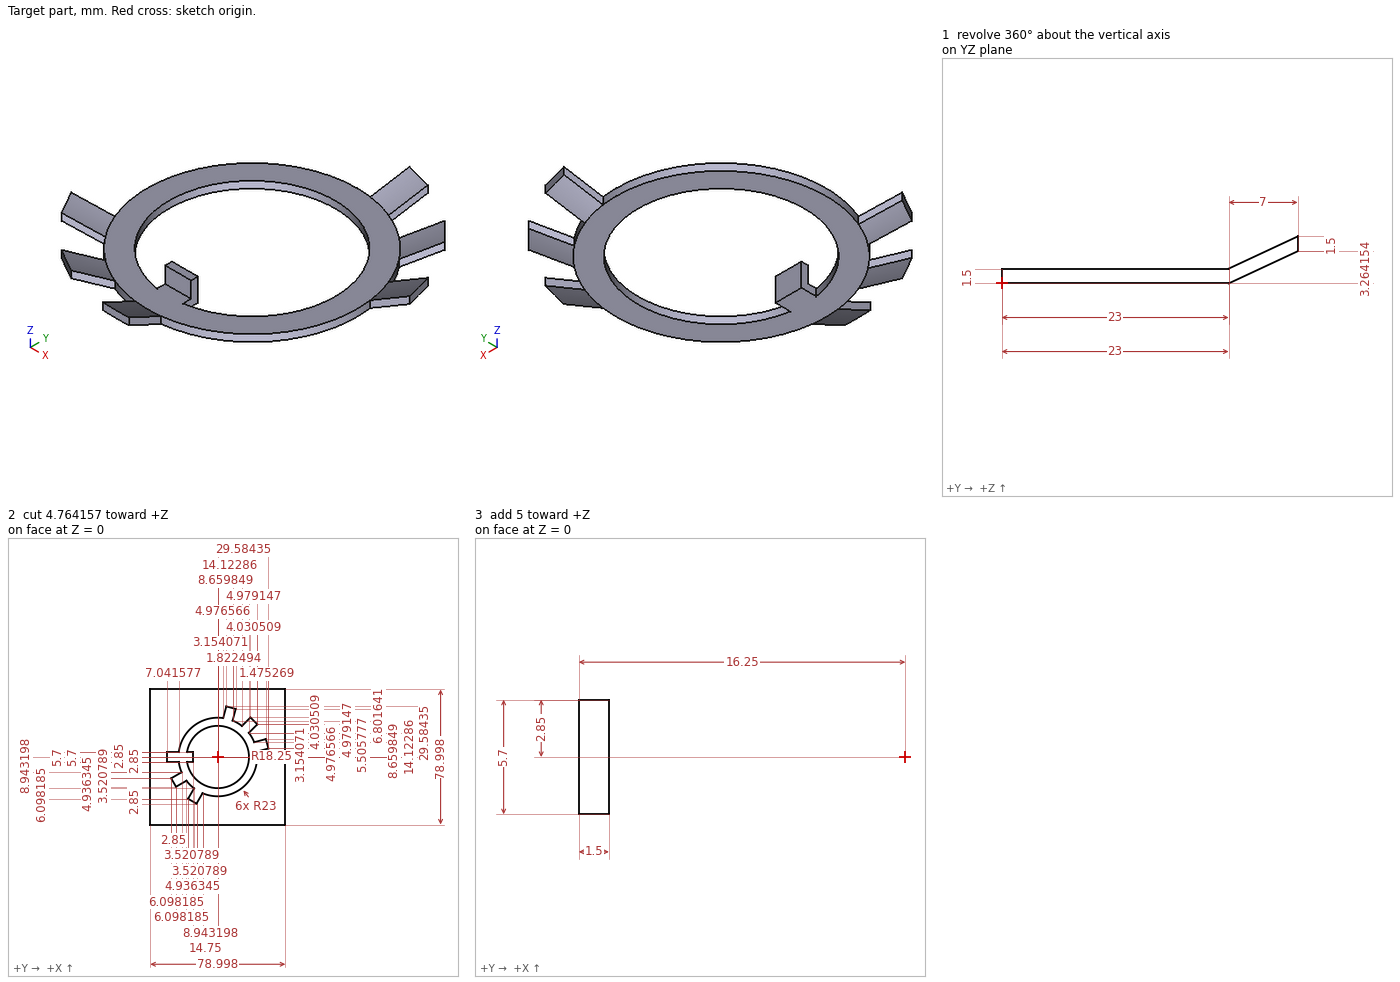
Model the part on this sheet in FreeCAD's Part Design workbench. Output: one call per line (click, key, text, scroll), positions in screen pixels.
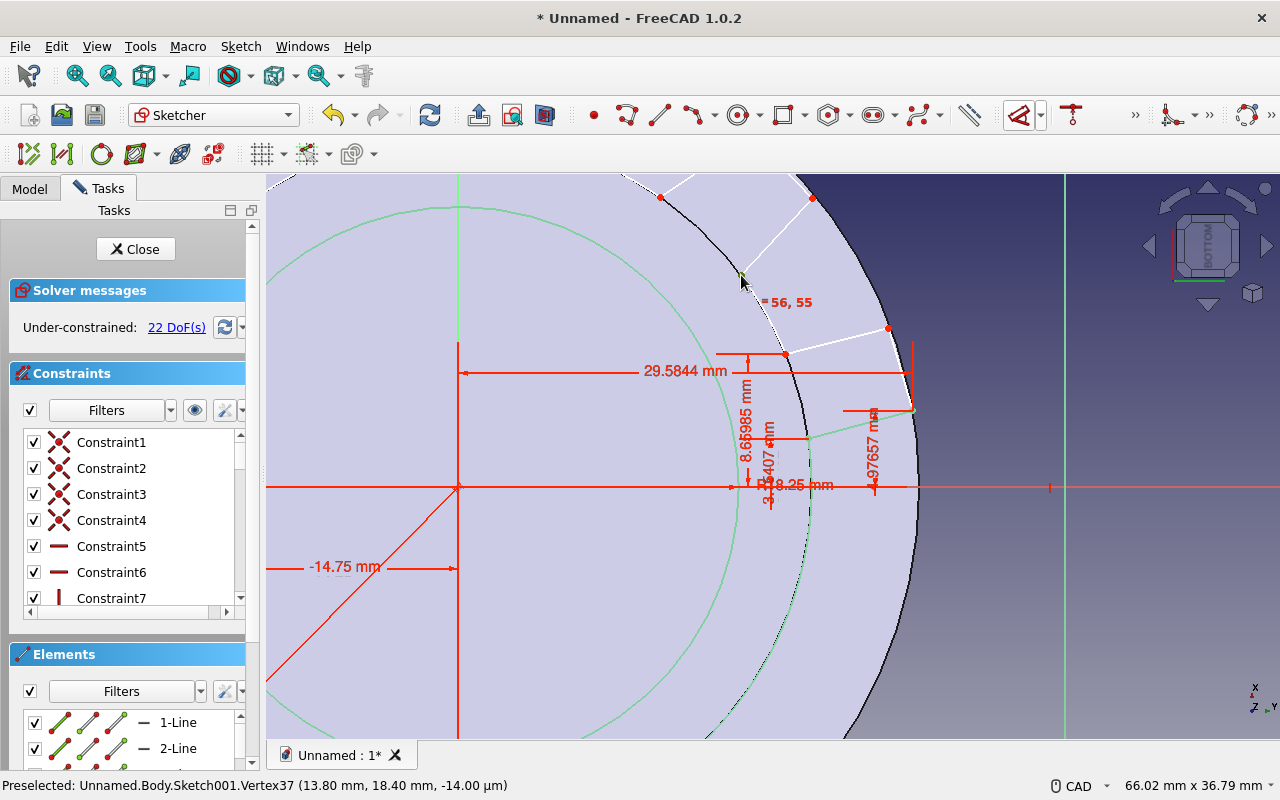
click(1040, 116)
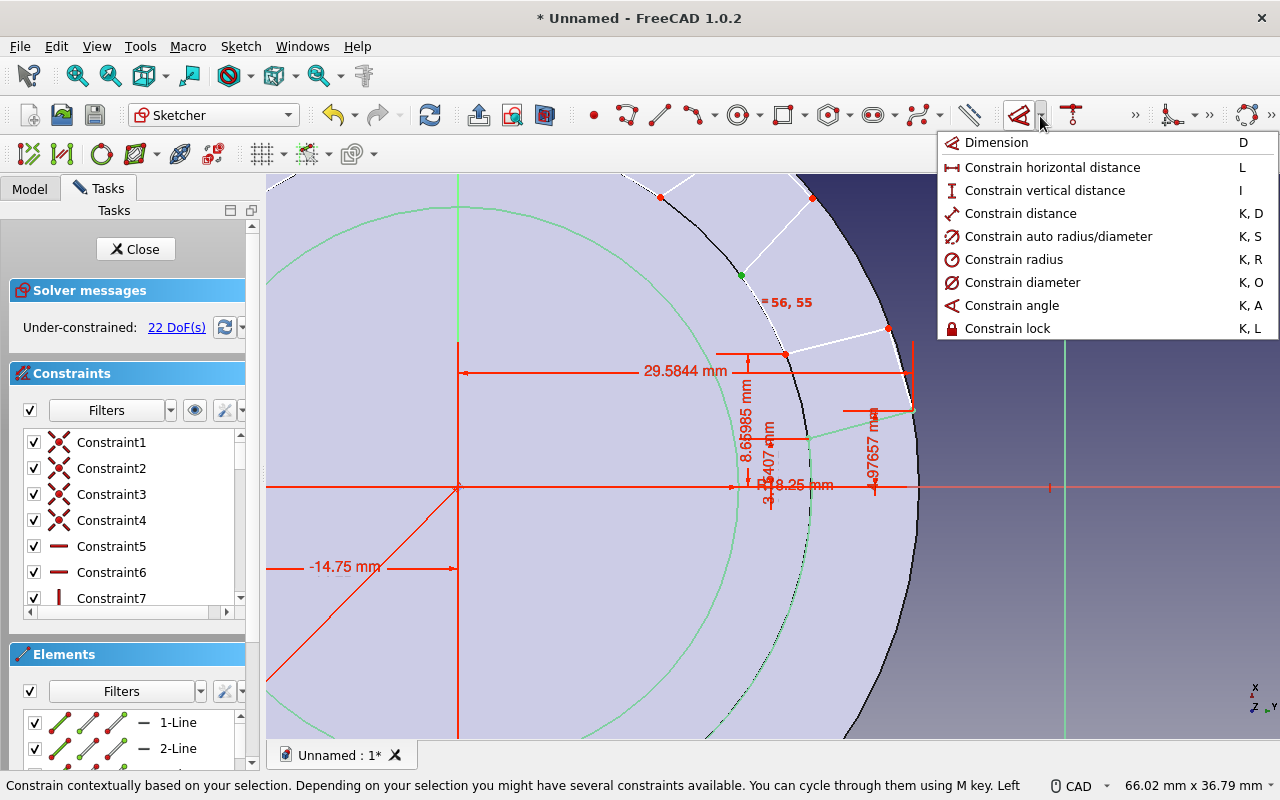
click(1108, 190)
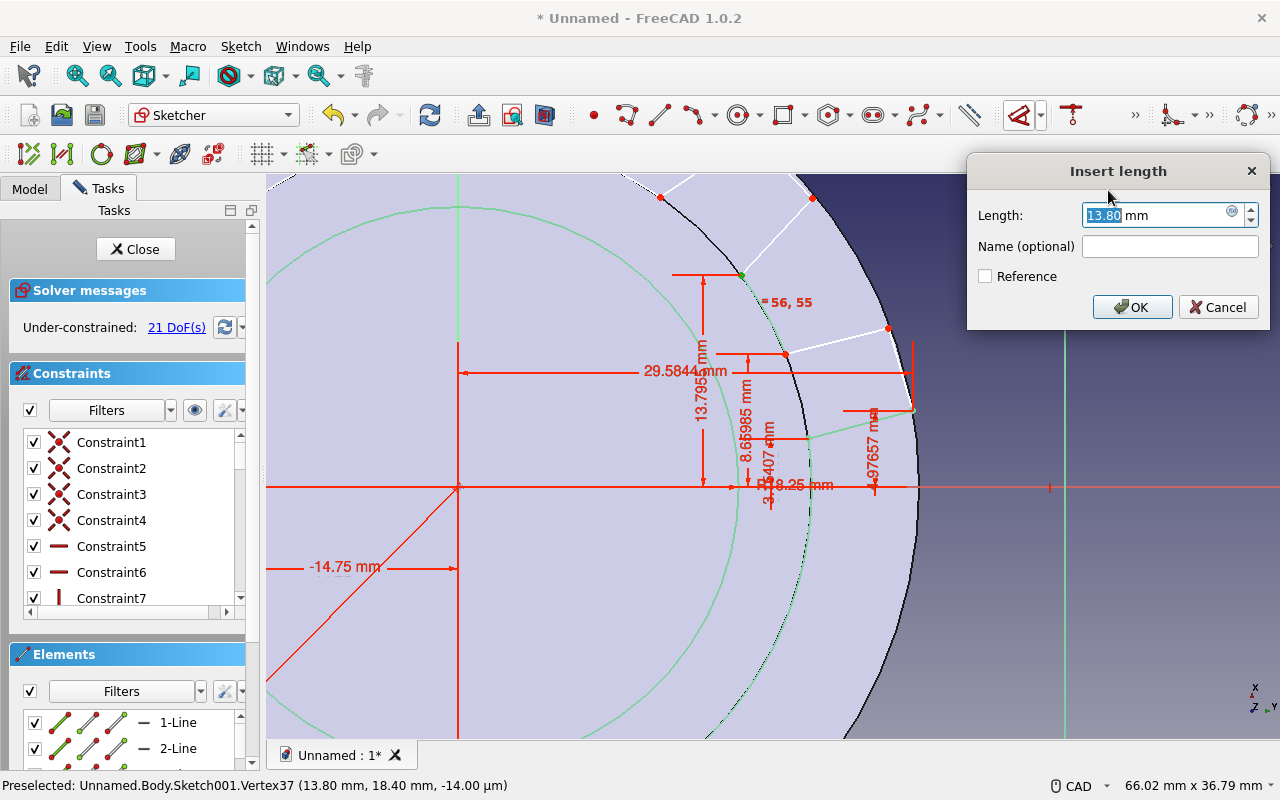
text(14.12286)
key(Return)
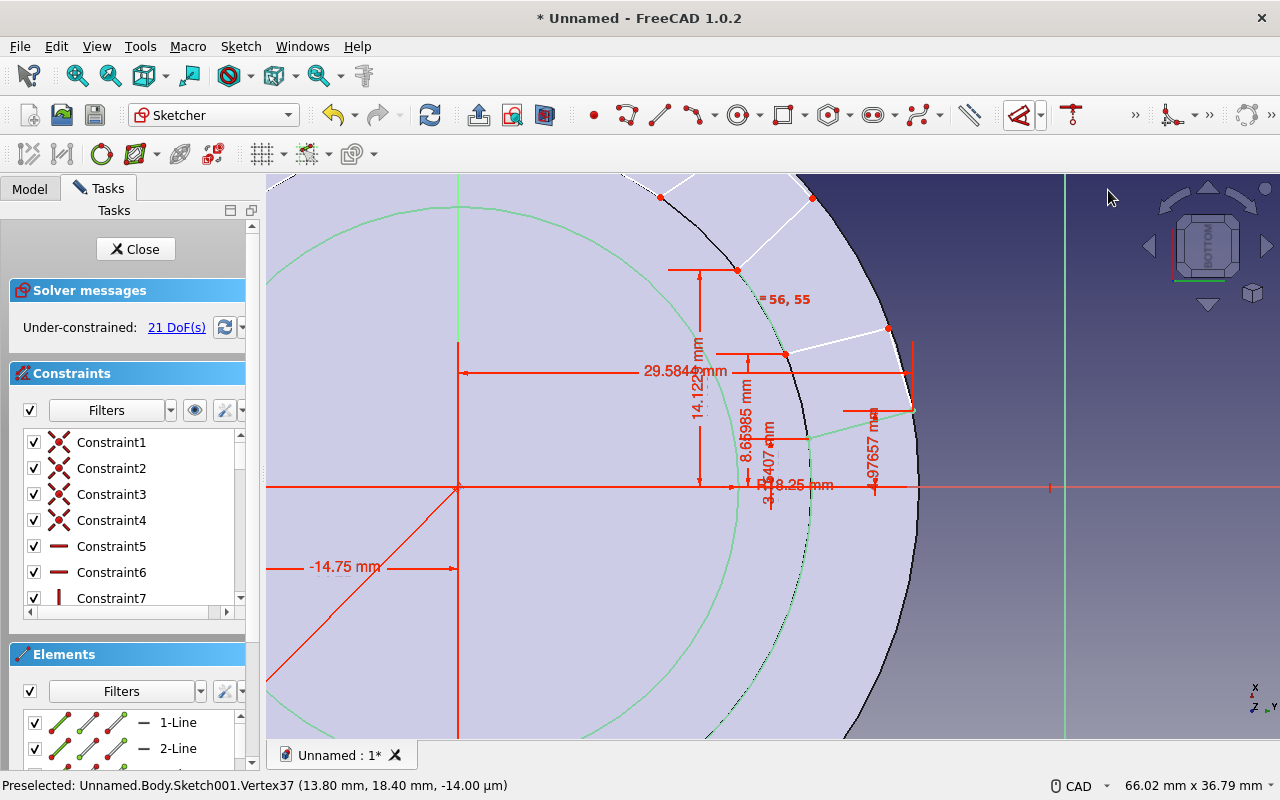
scroll(811, 443, down, 6)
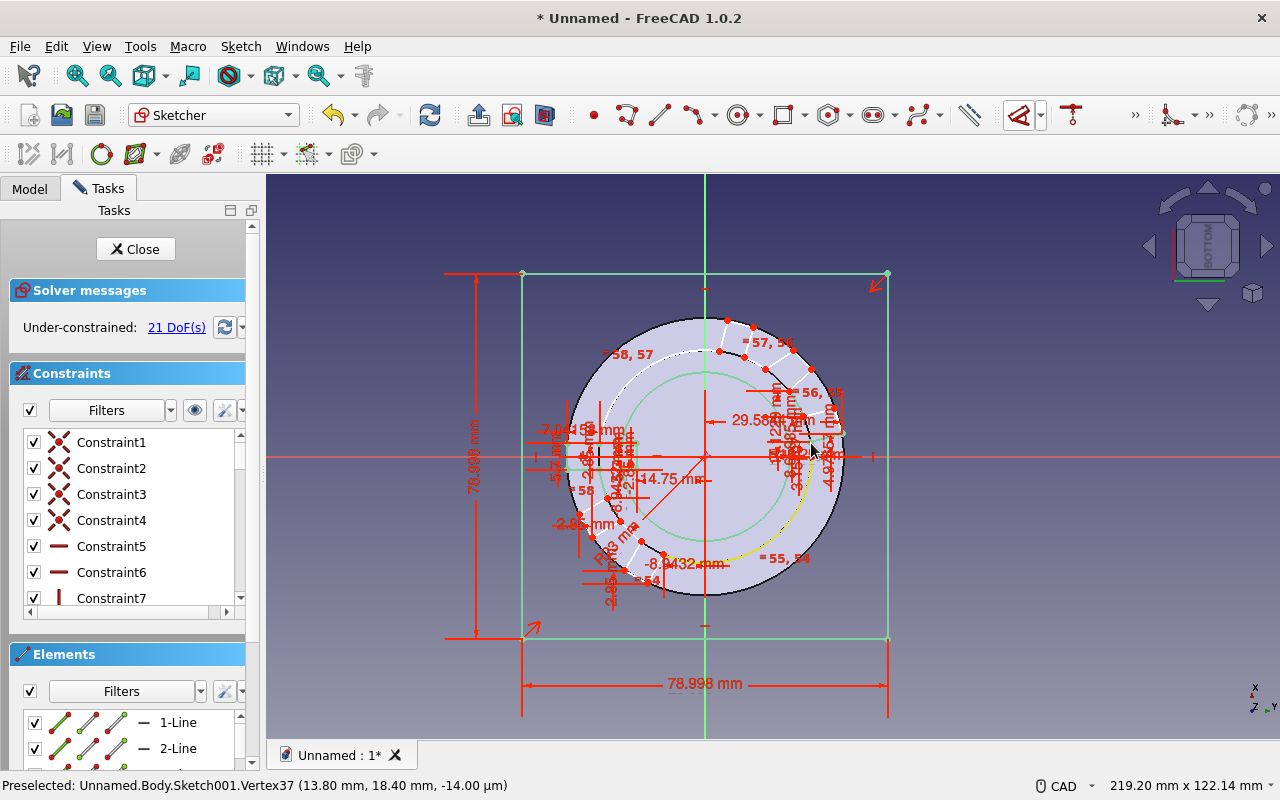
click(766, 369)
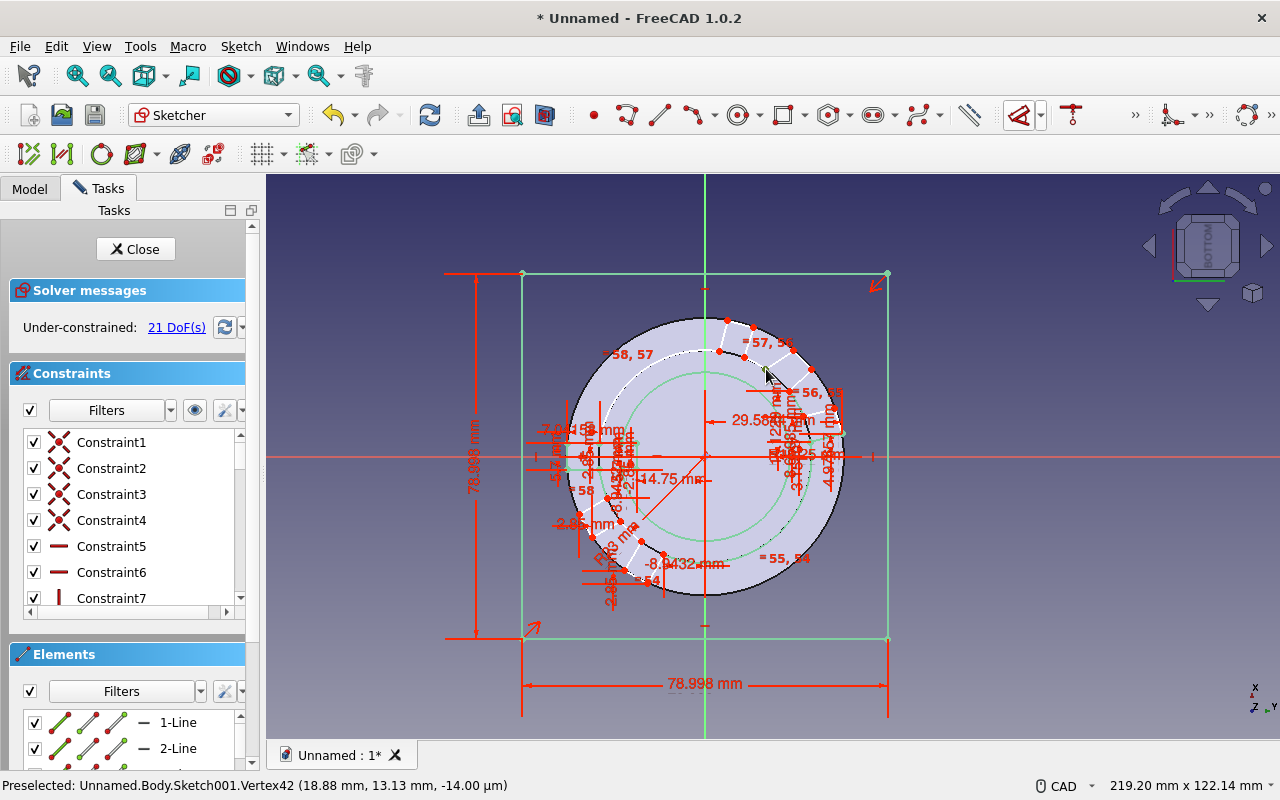
click(1040, 116)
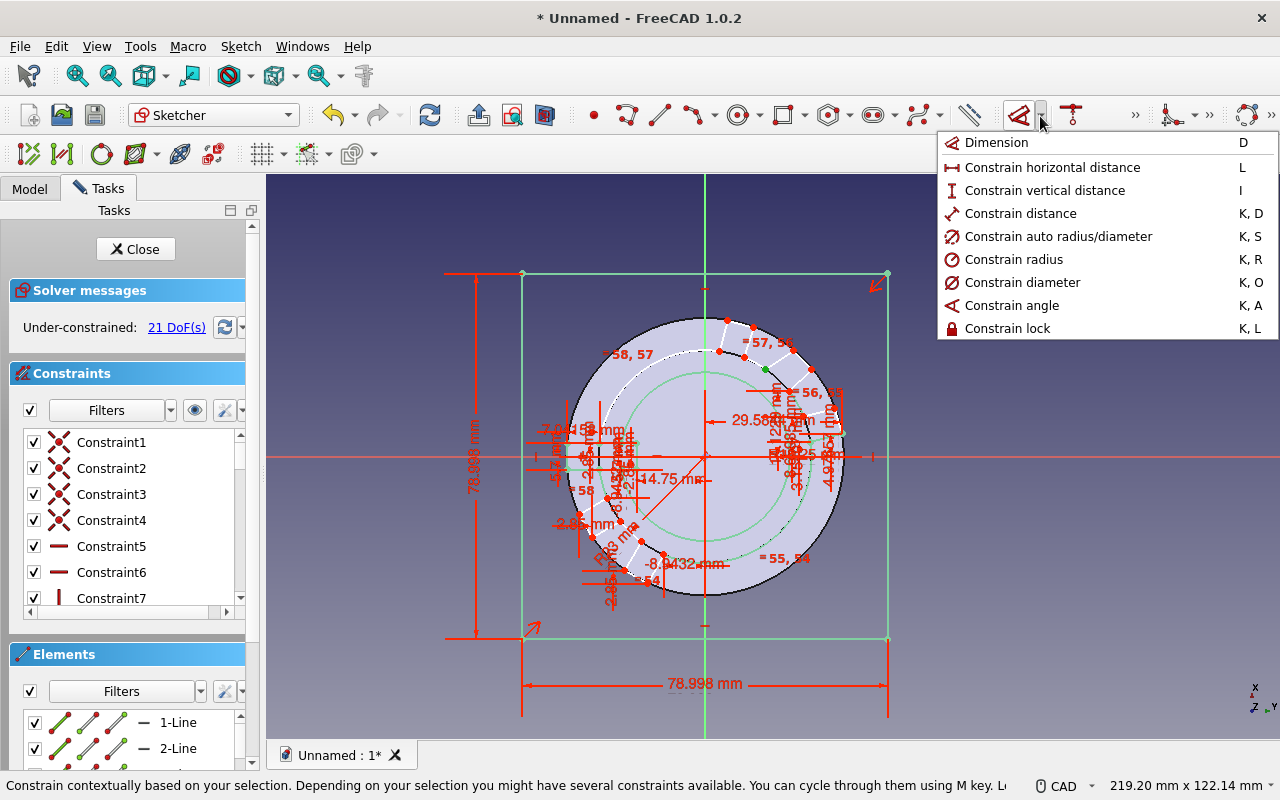
click(1108, 168)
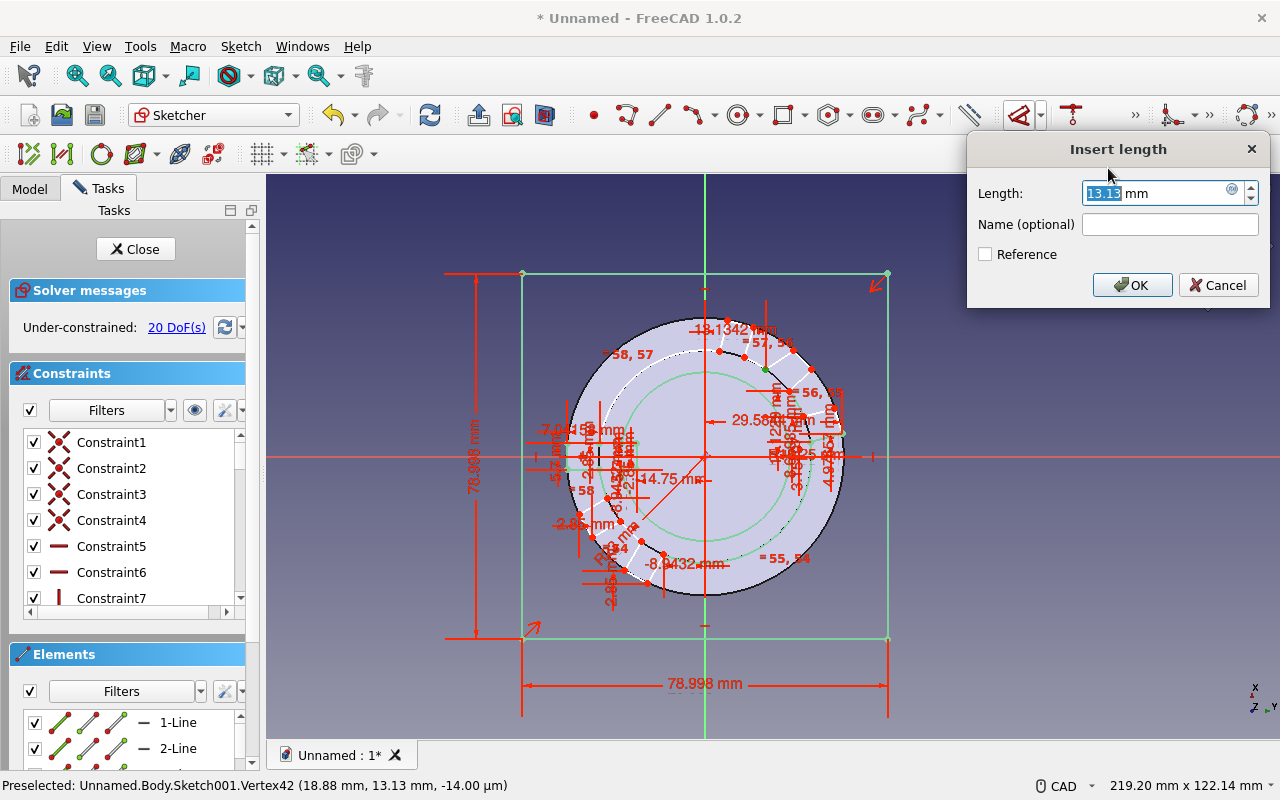
text(14.12286)
key(Return)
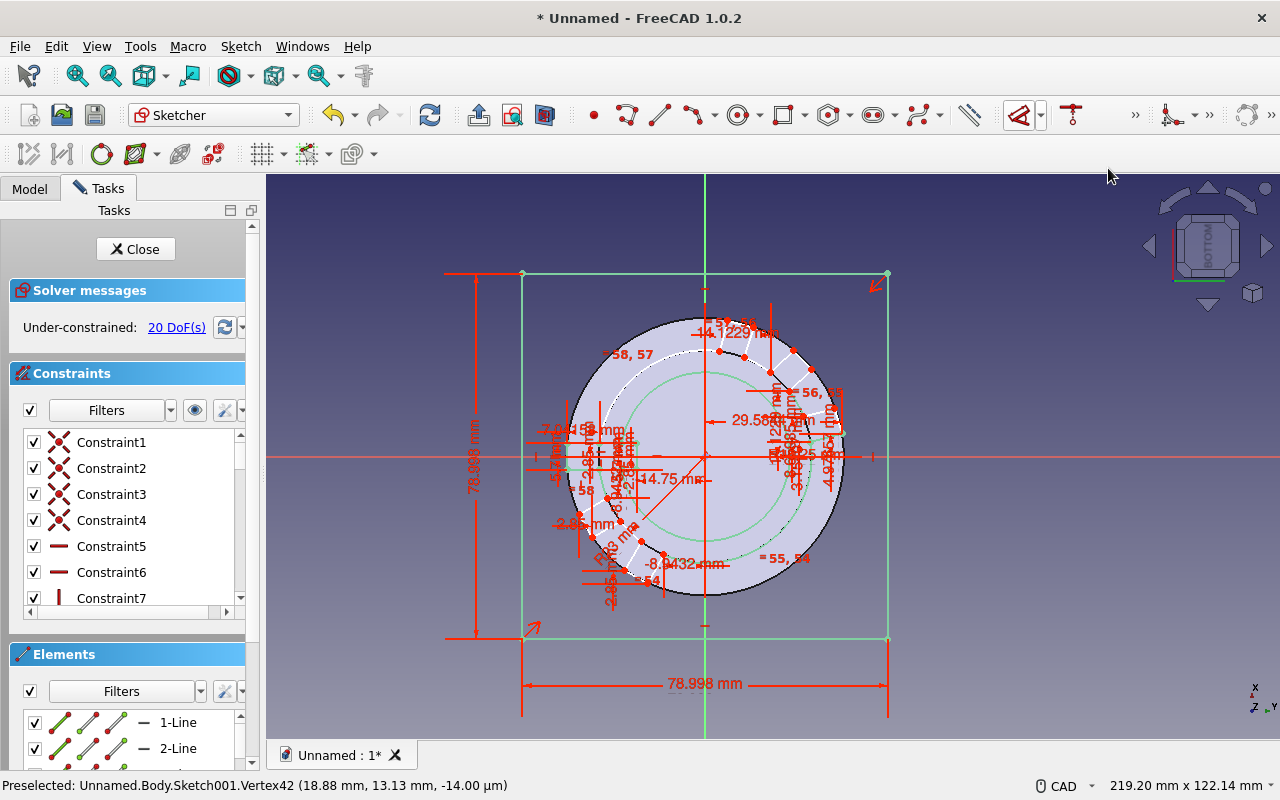
click(744, 358)